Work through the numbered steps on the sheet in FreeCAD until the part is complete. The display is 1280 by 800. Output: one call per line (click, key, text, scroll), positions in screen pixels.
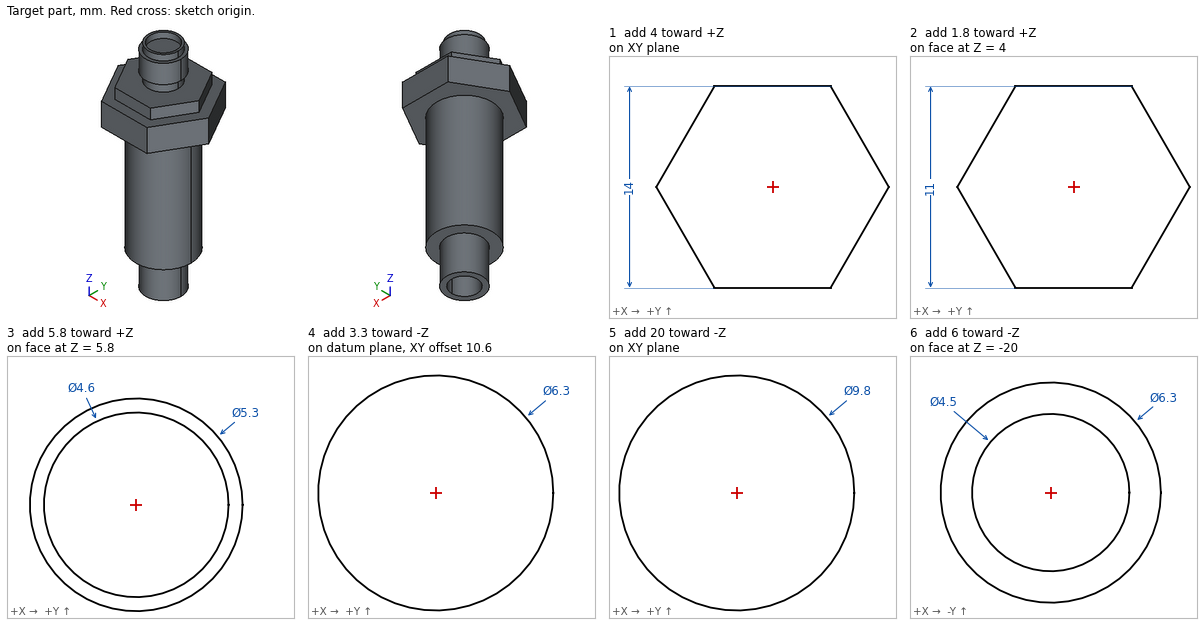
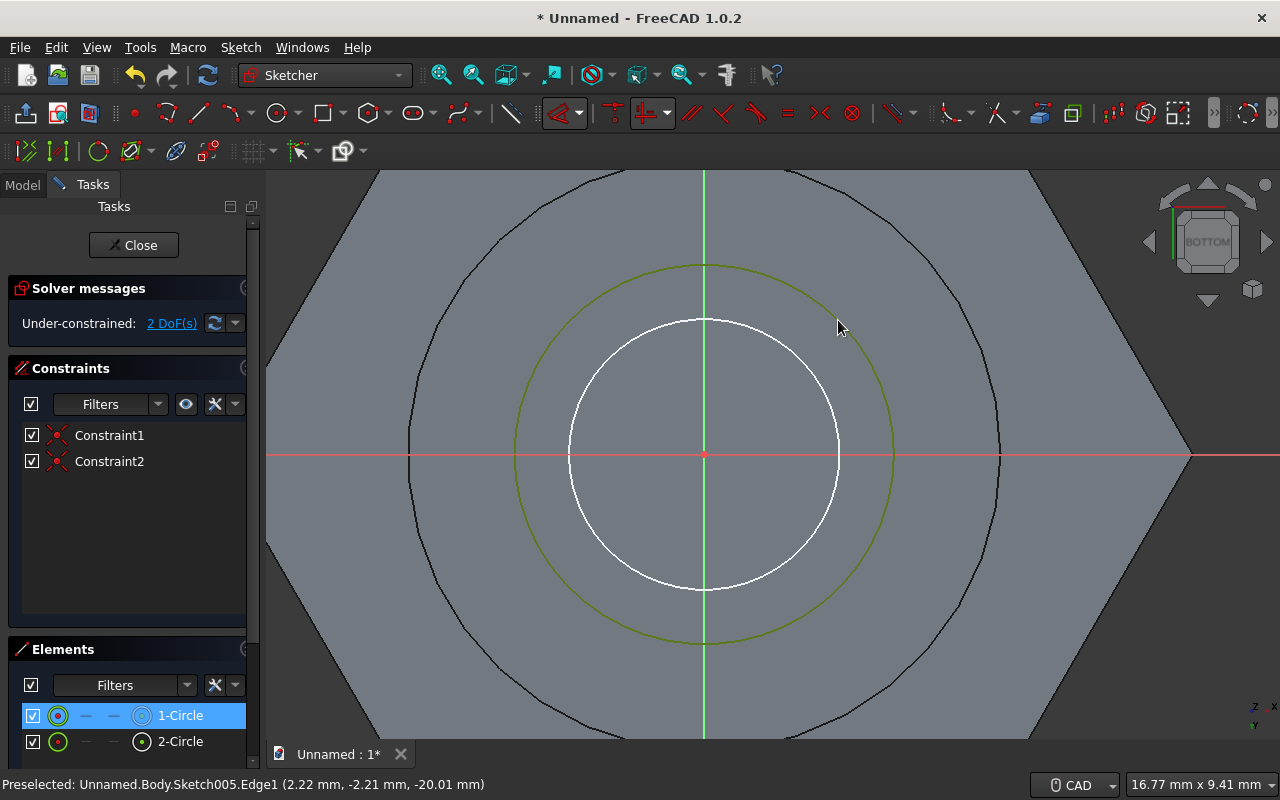
click(582, 114)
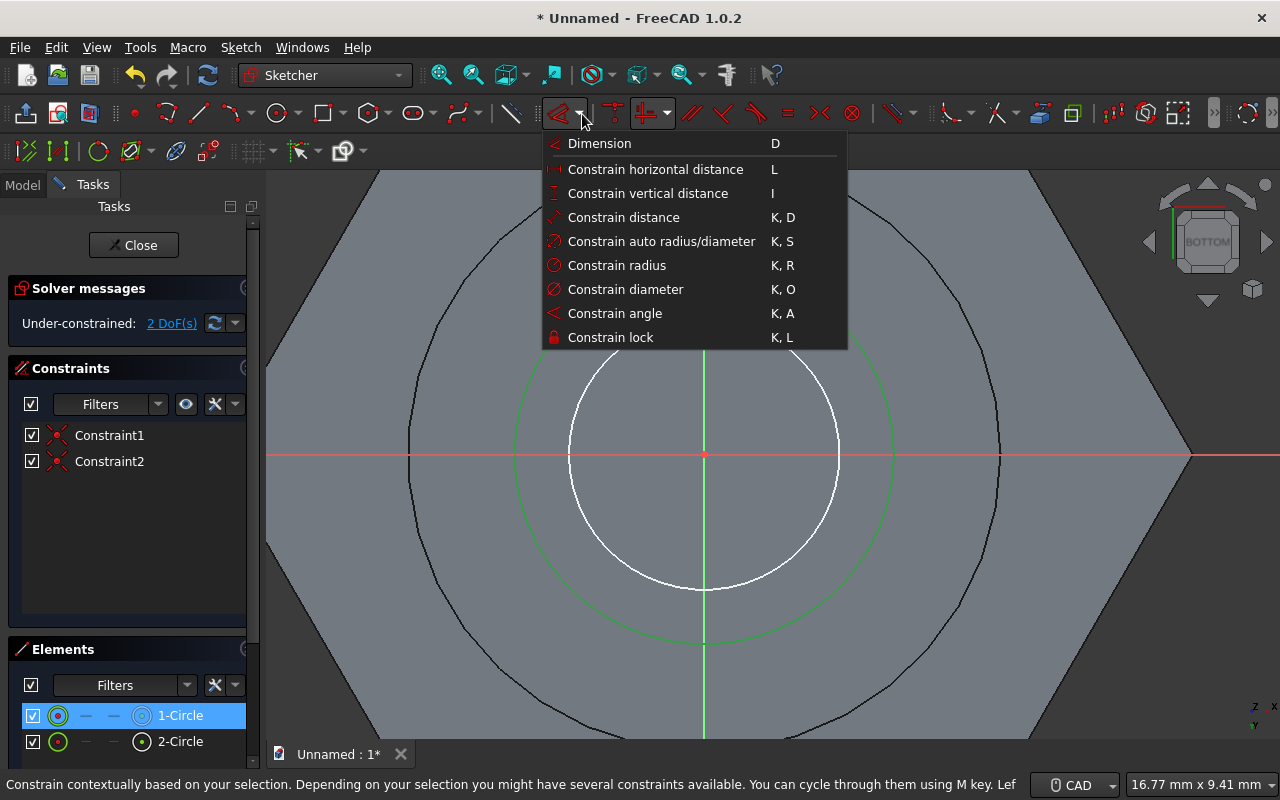
click(695, 289)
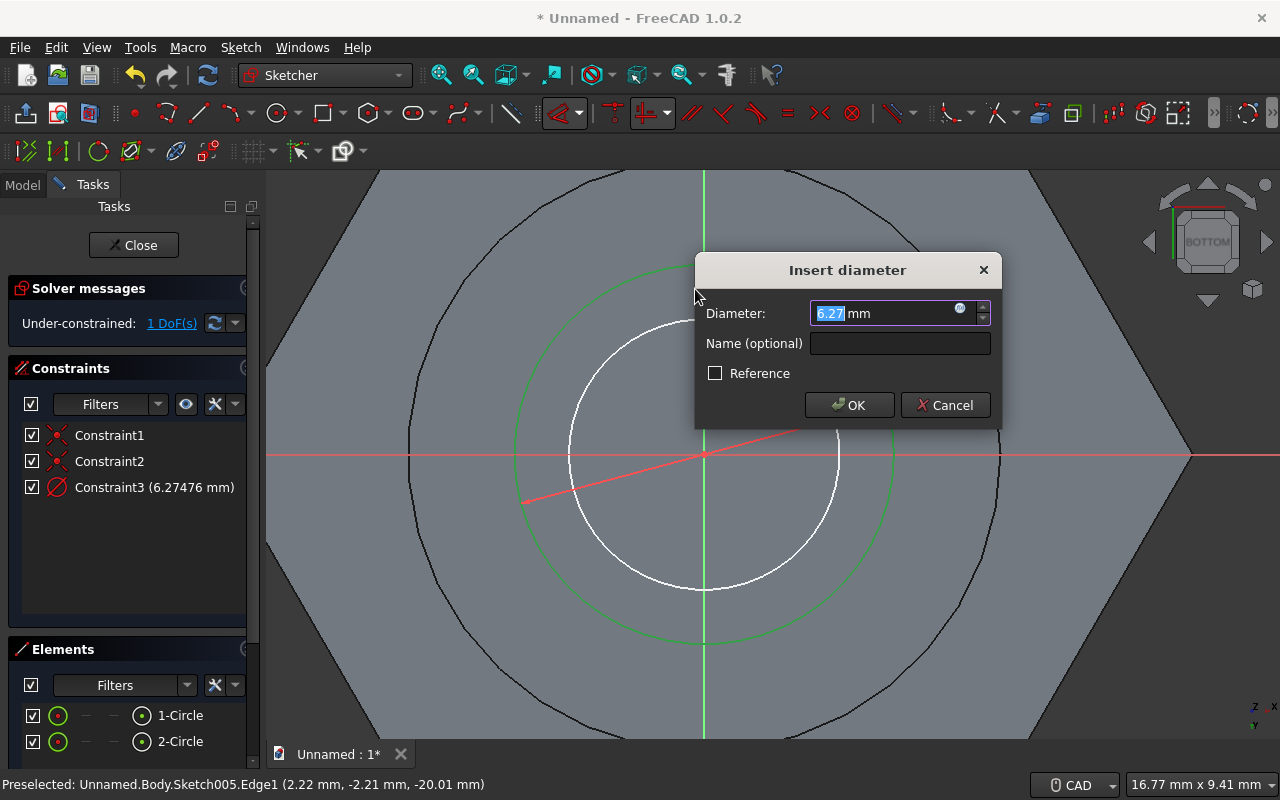
text(6.3)
key(Return)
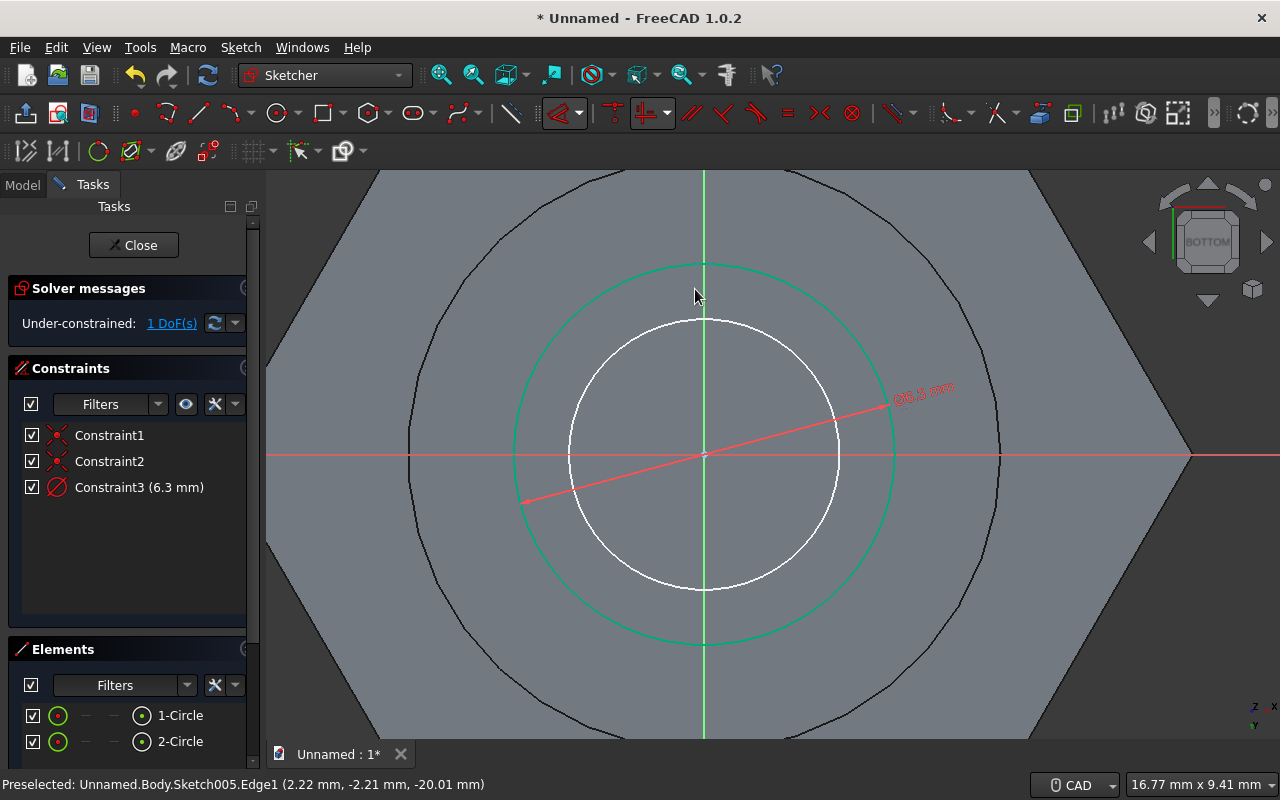
click(800, 359)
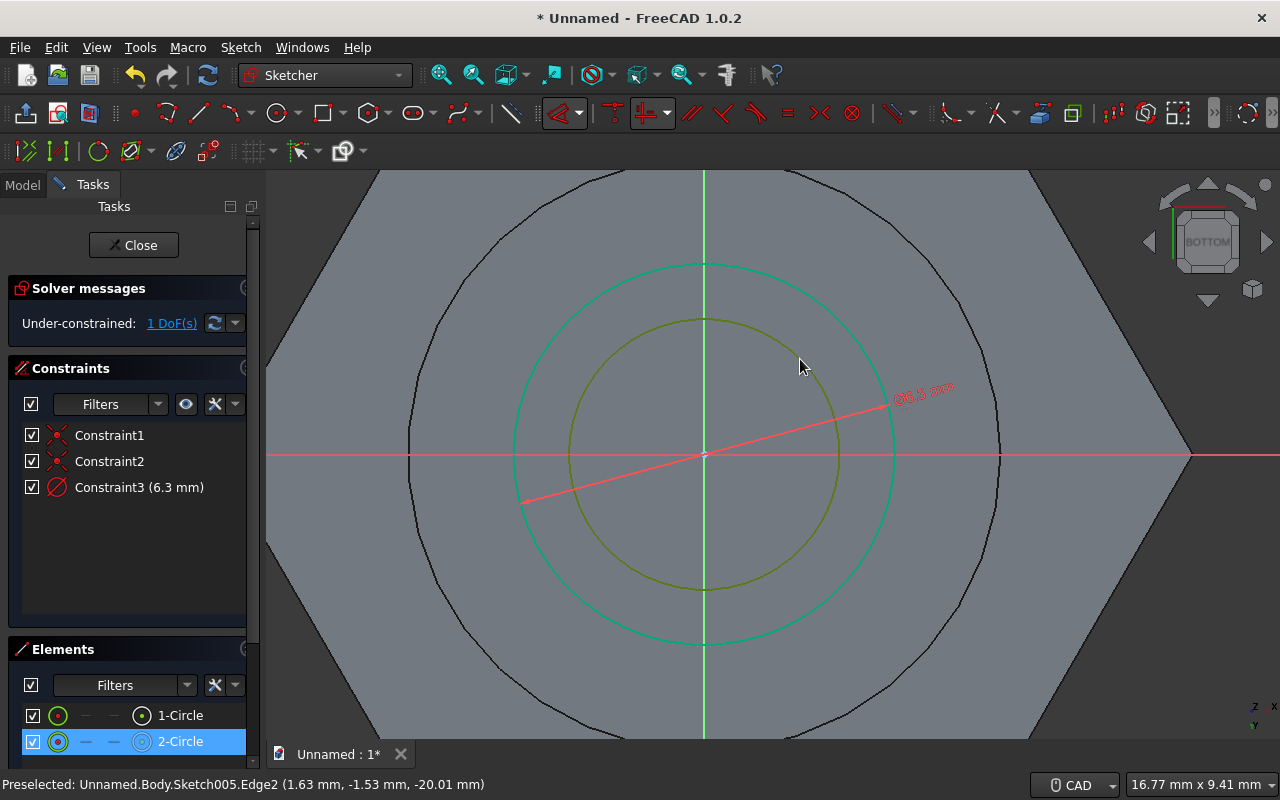
key(k)
key(o)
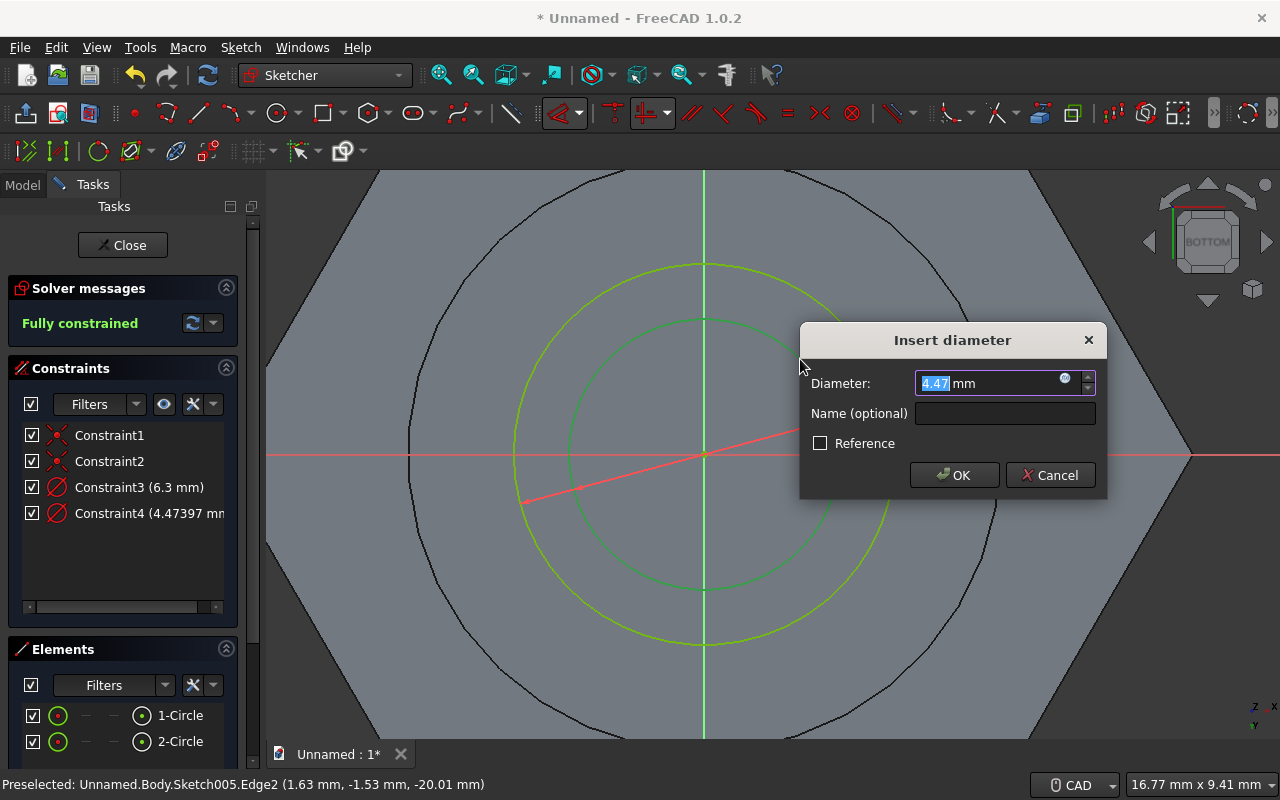
text(4.5)
key(Return)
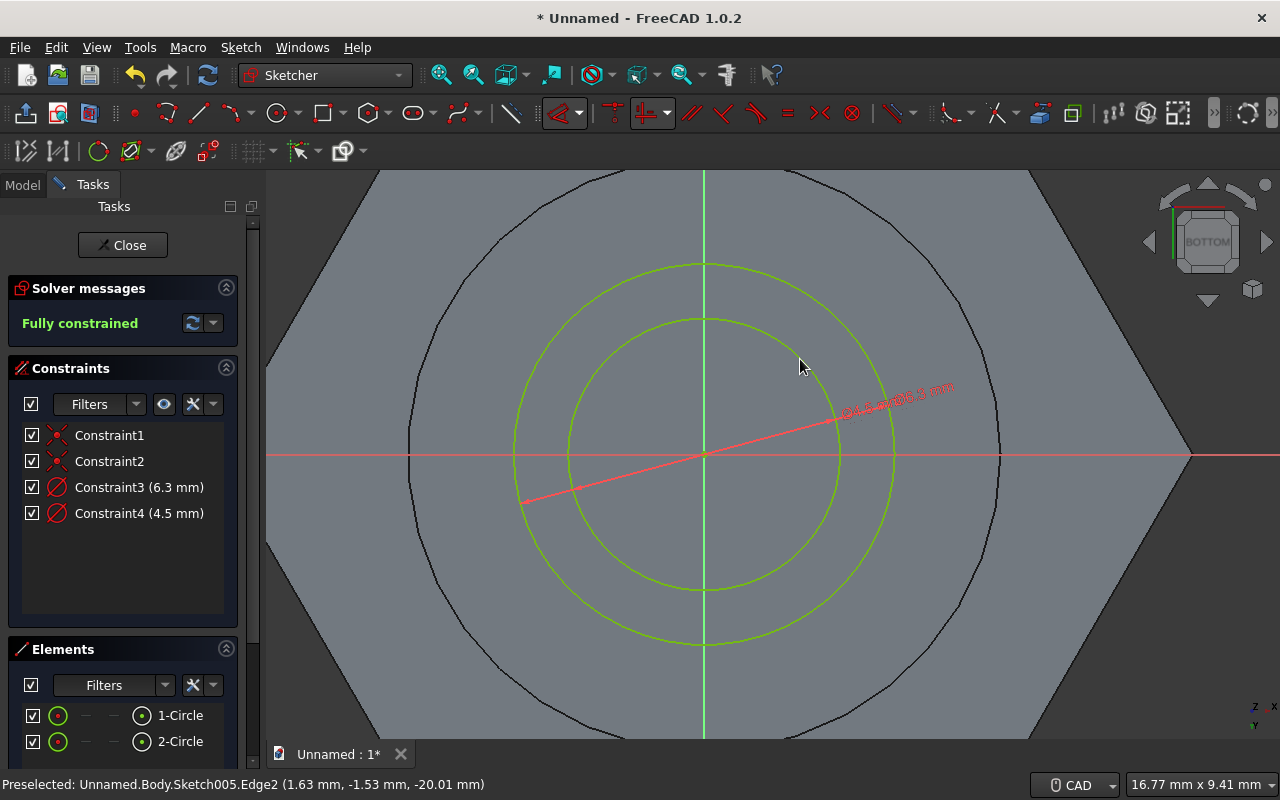
click(123, 245)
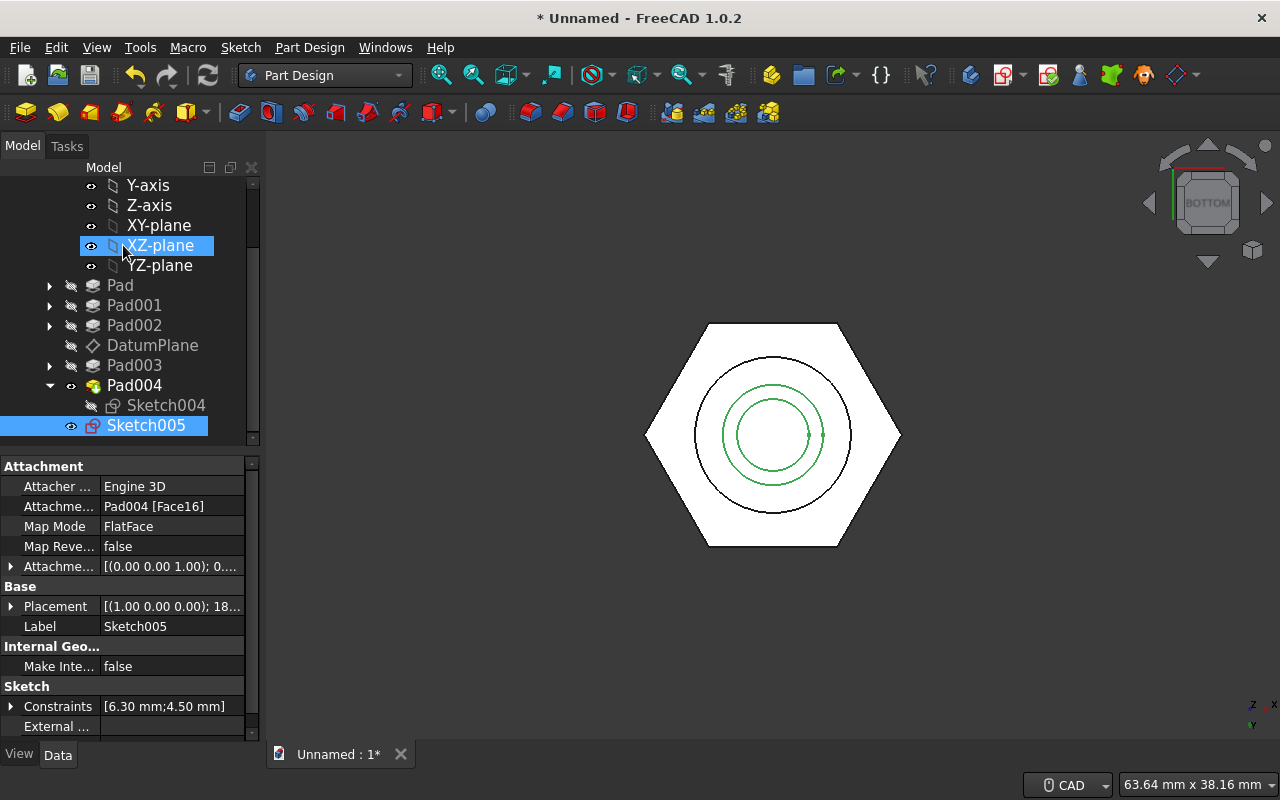
click(26, 112)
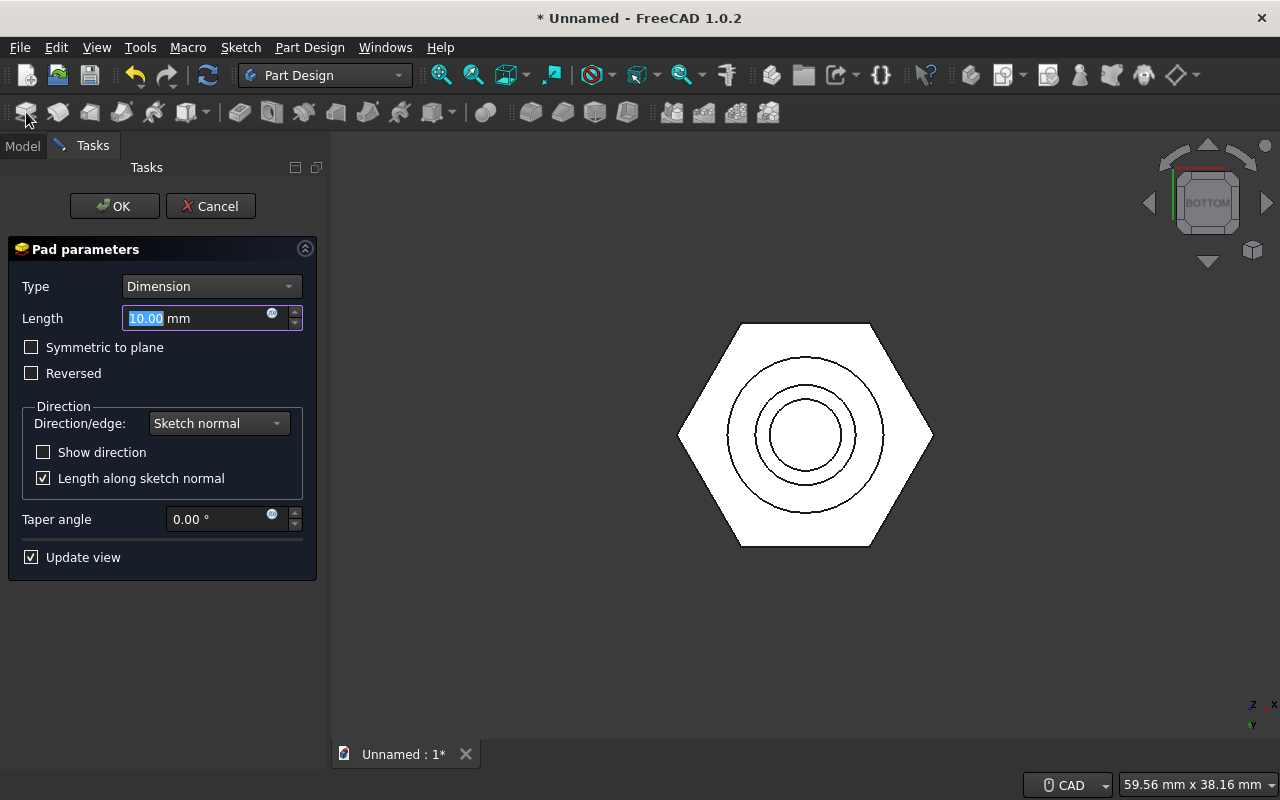
text(6)
key(Tab)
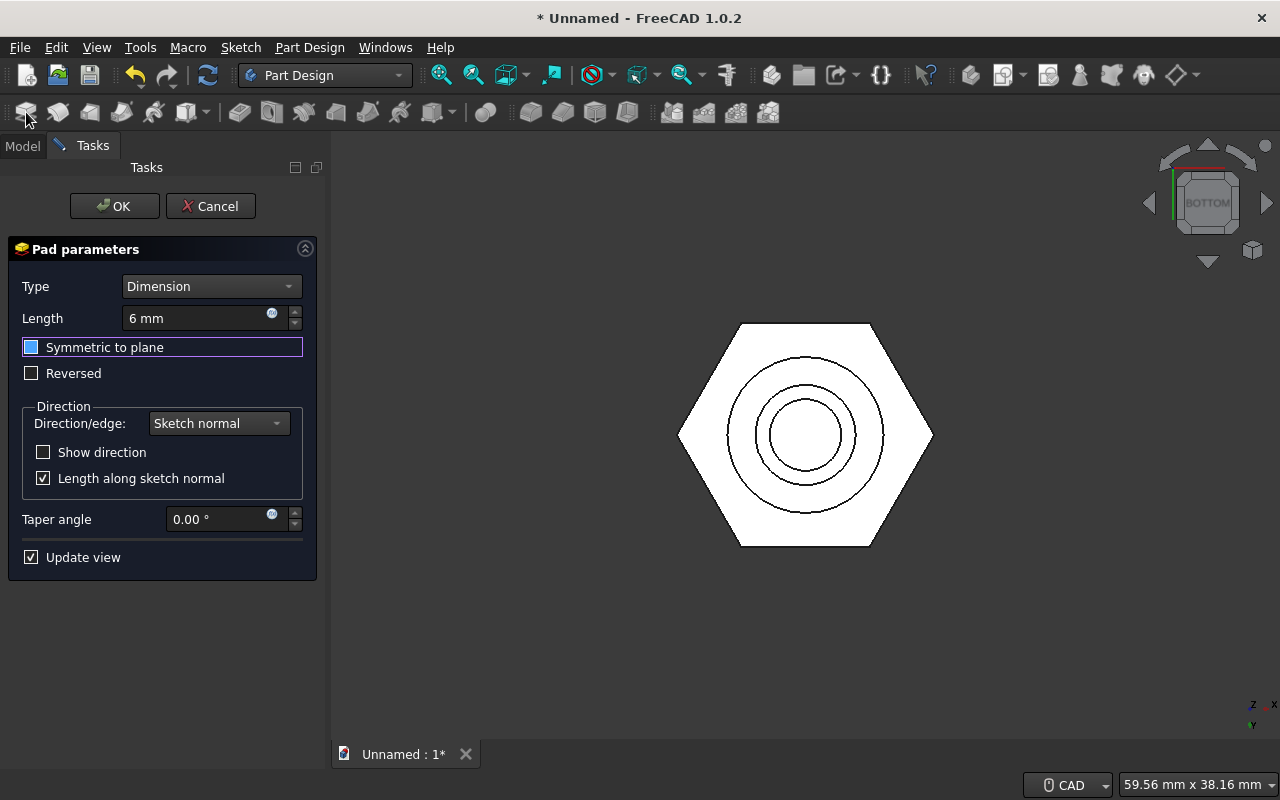
click(115, 206)